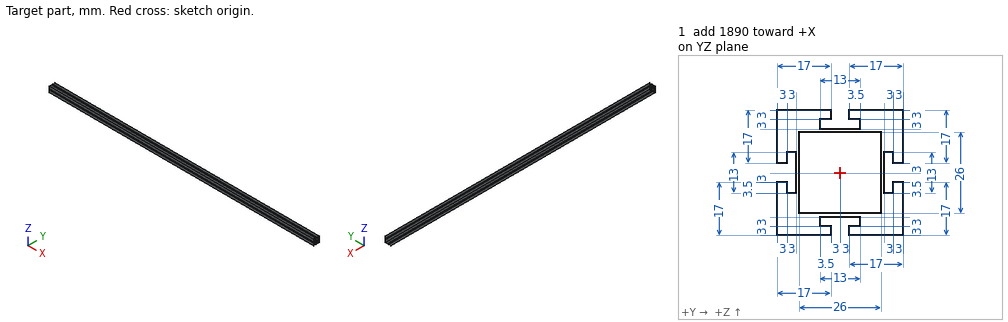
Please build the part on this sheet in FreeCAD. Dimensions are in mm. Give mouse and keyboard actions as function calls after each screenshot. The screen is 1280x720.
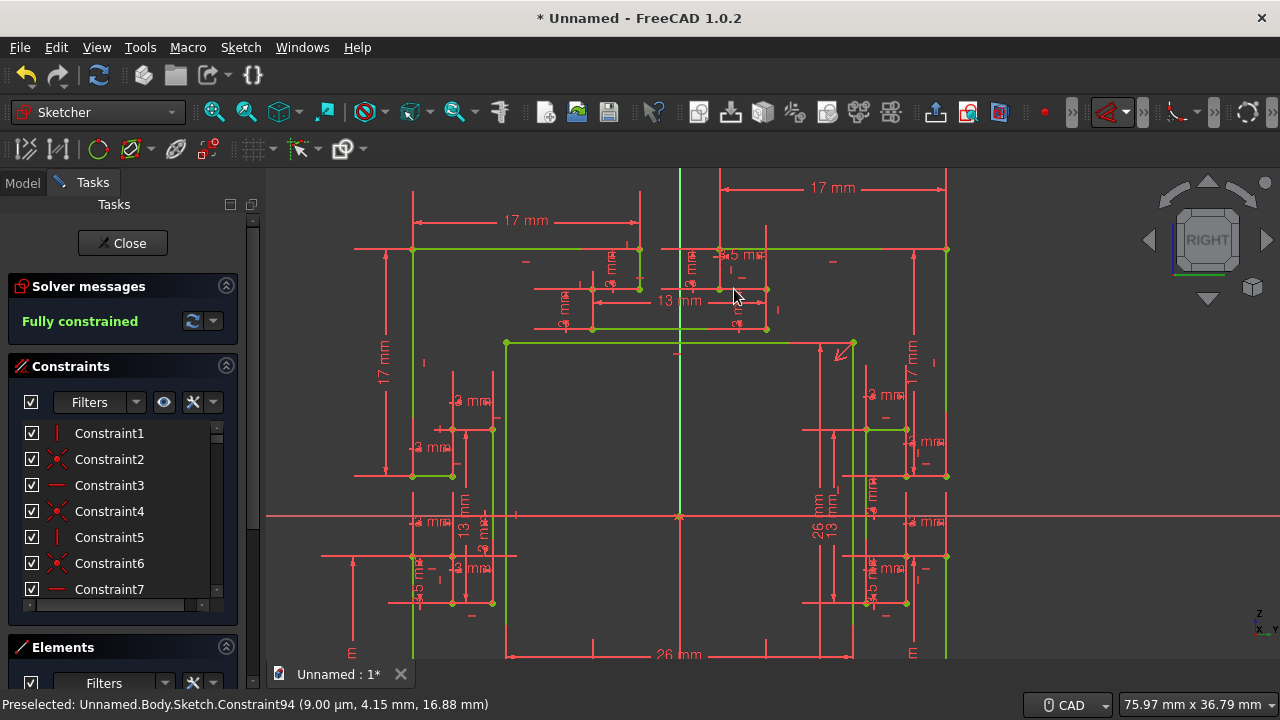
click(123, 243)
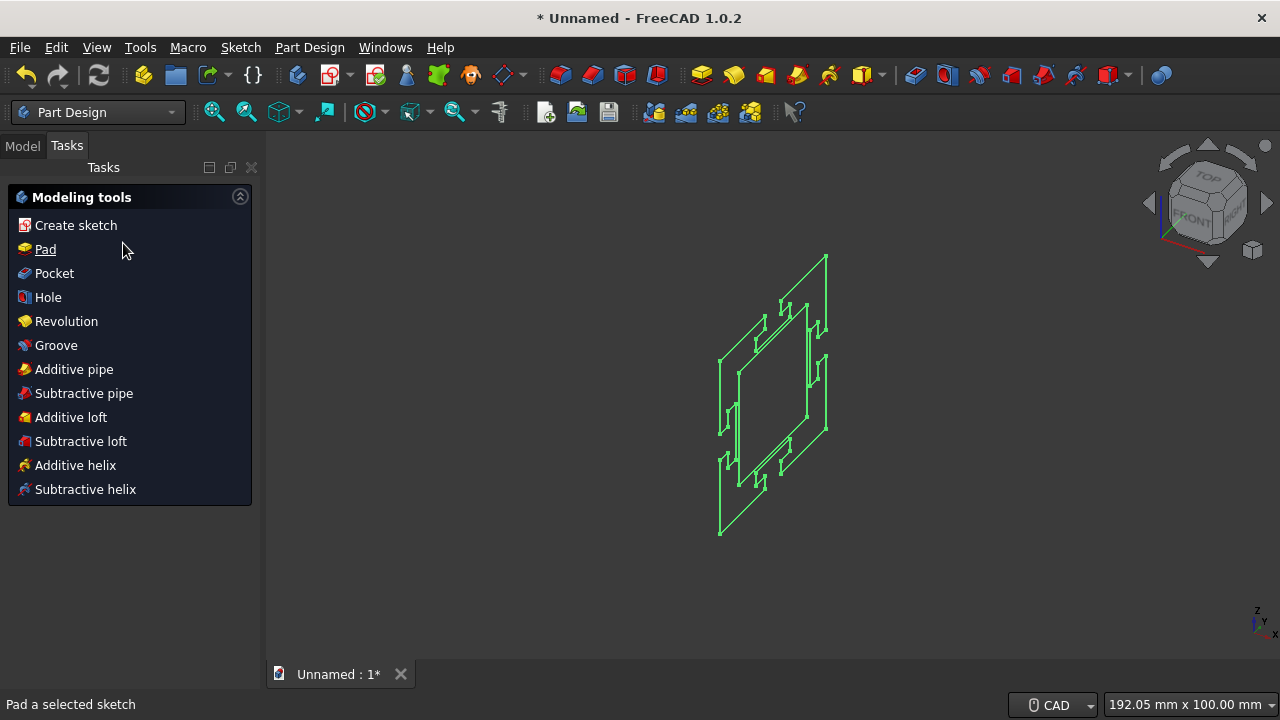
click(702, 76)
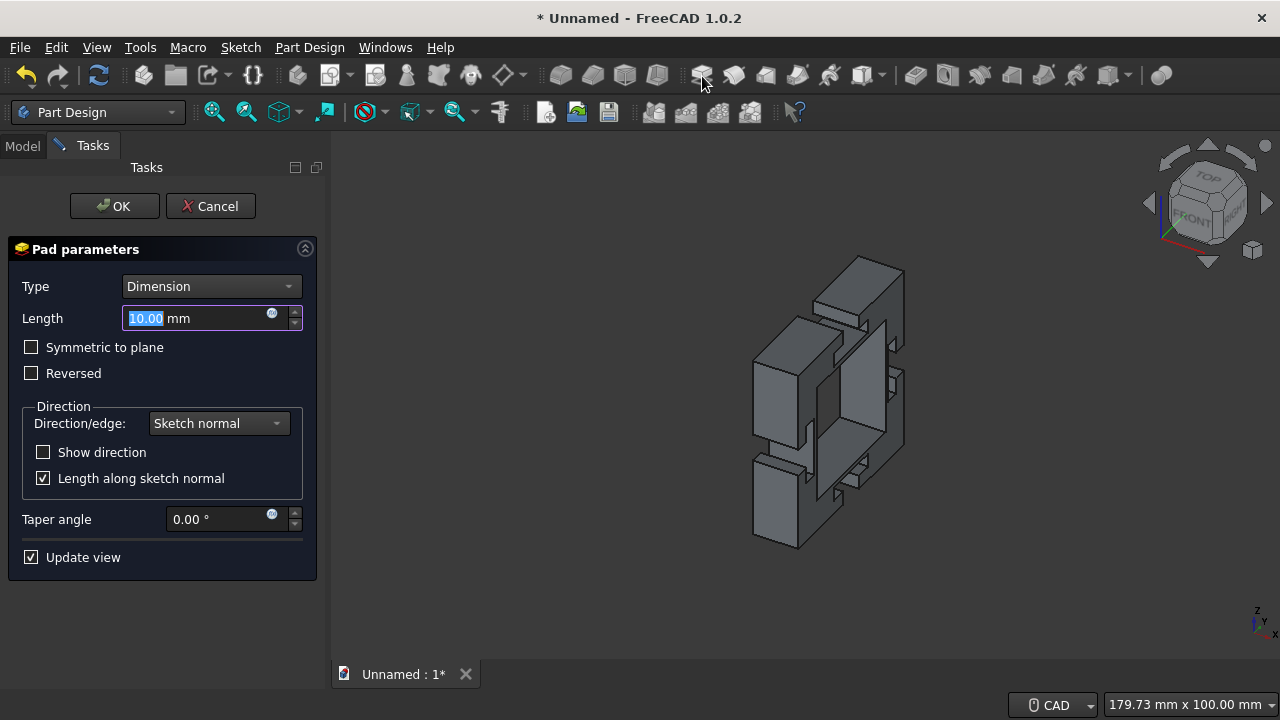
text(1890)
key(Tab)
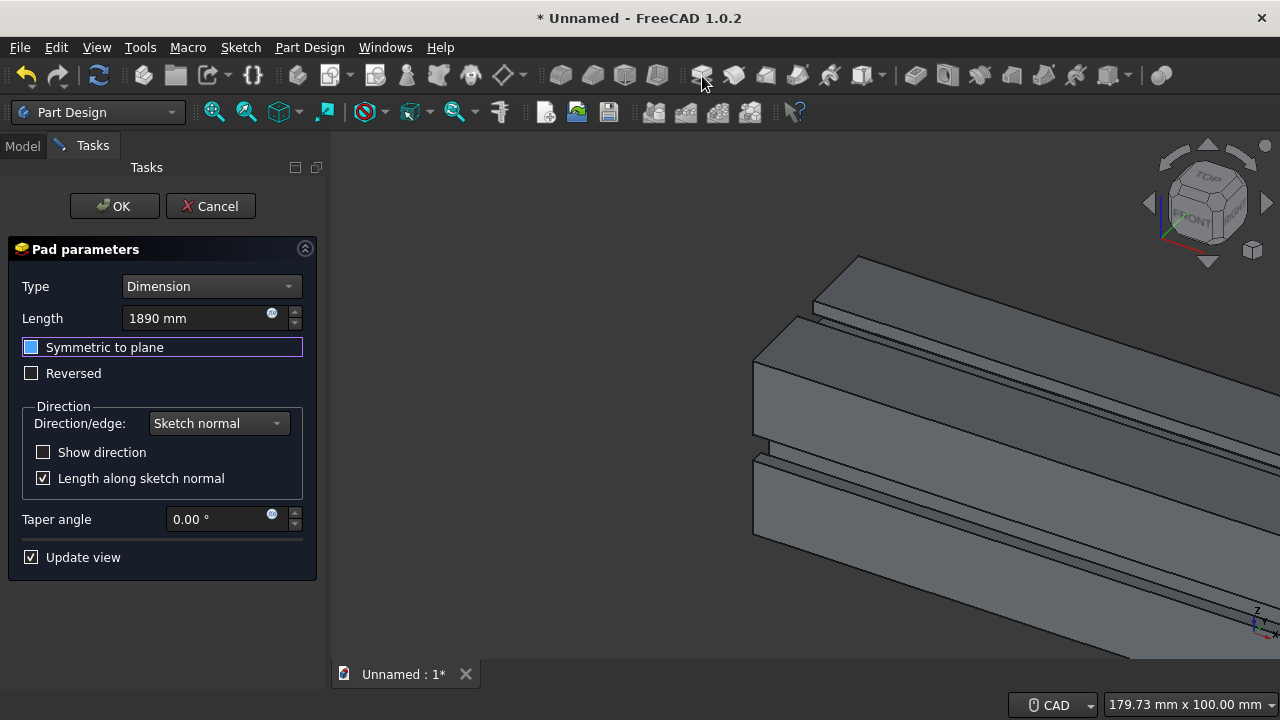
click(115, 206)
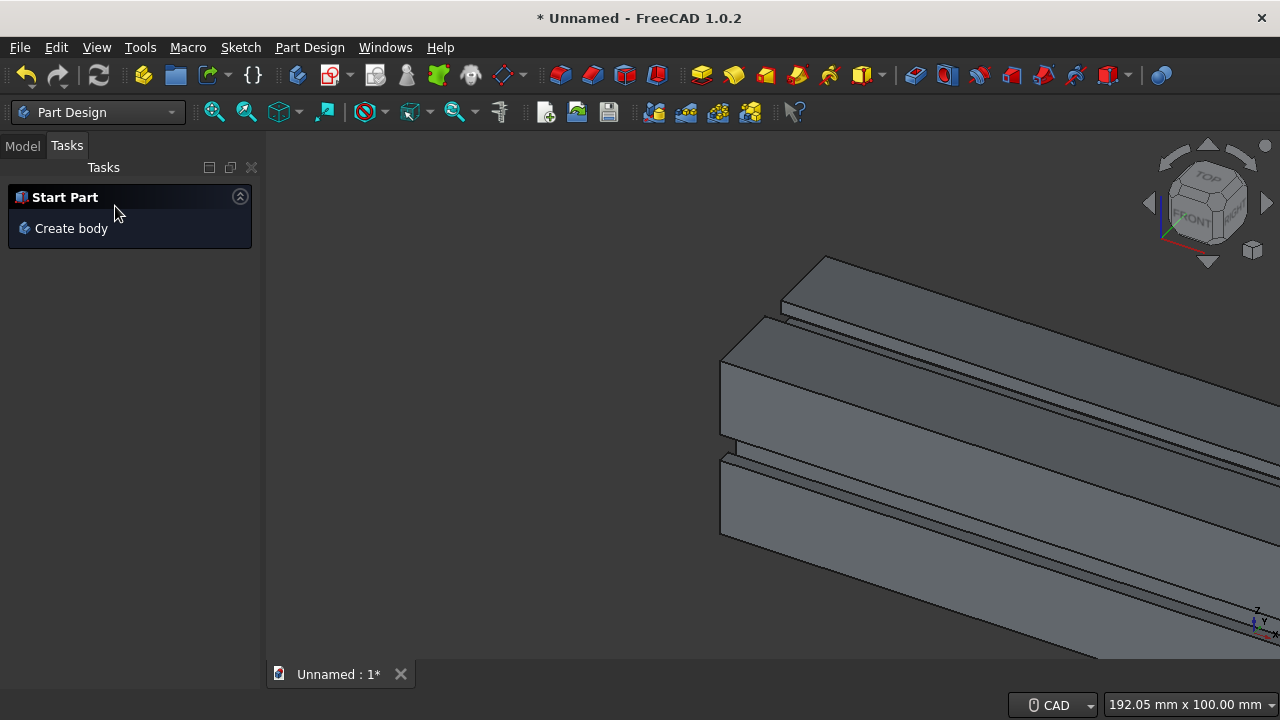
key(0)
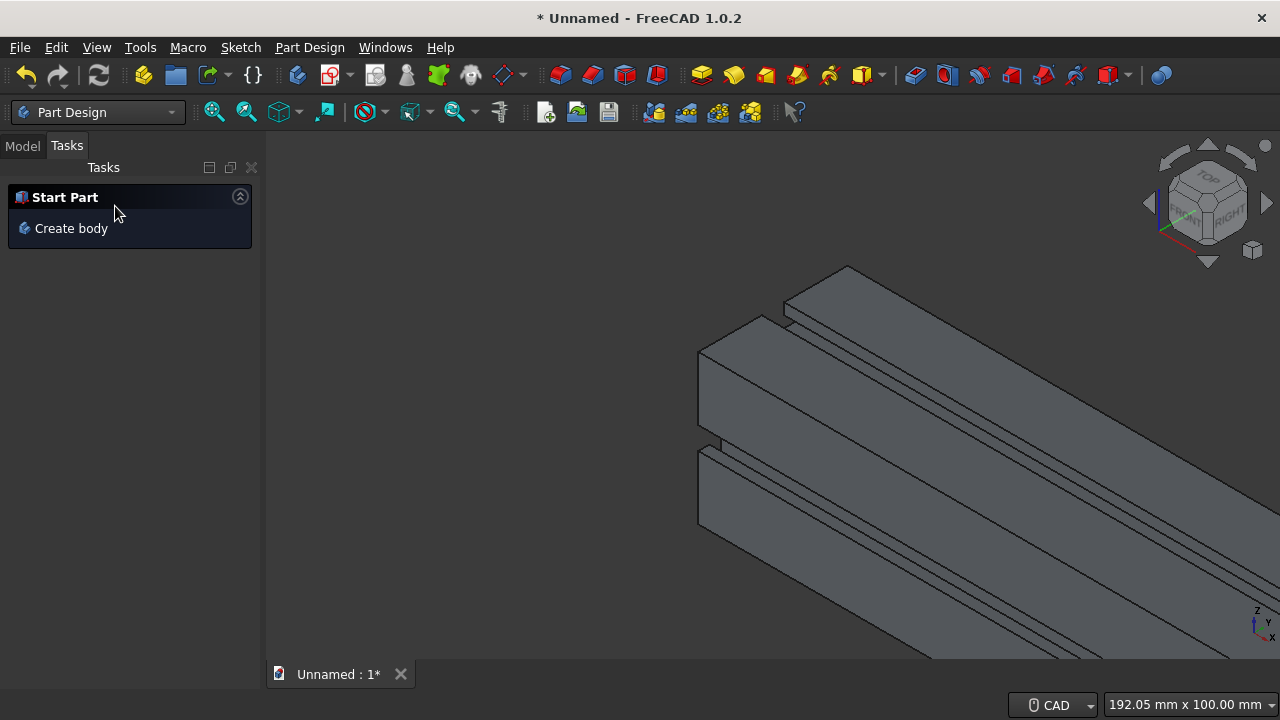
click(216, 112)